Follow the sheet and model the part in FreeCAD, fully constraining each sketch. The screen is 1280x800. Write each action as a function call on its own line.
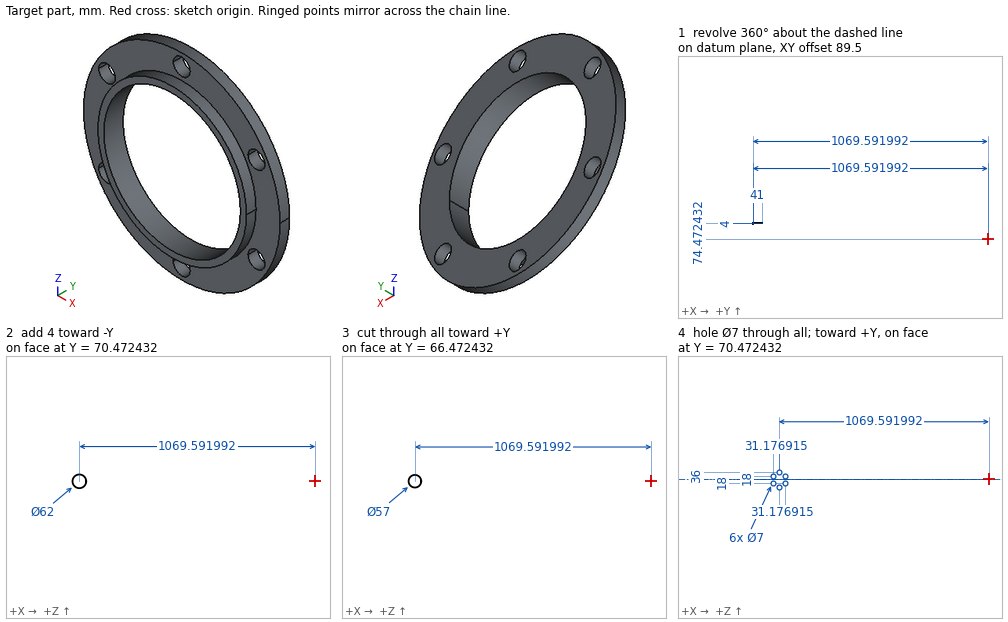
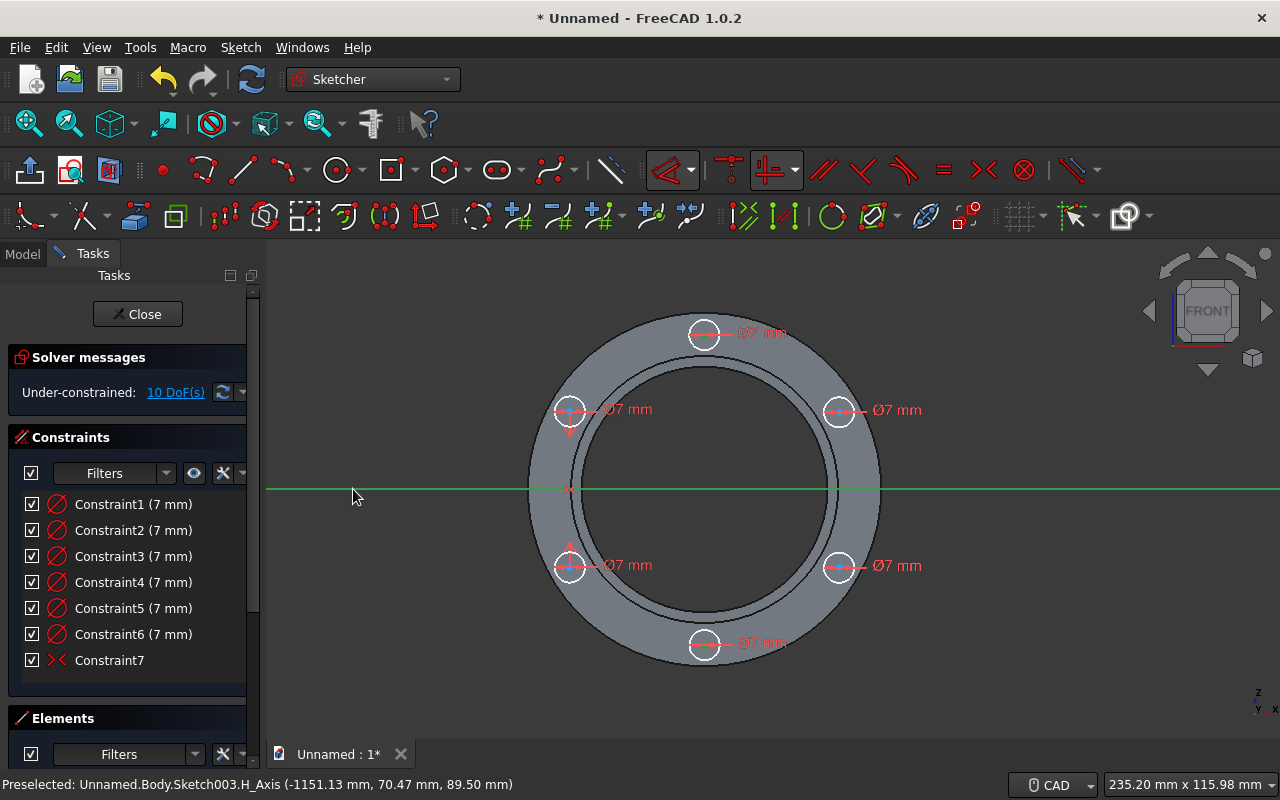
click(984, 170)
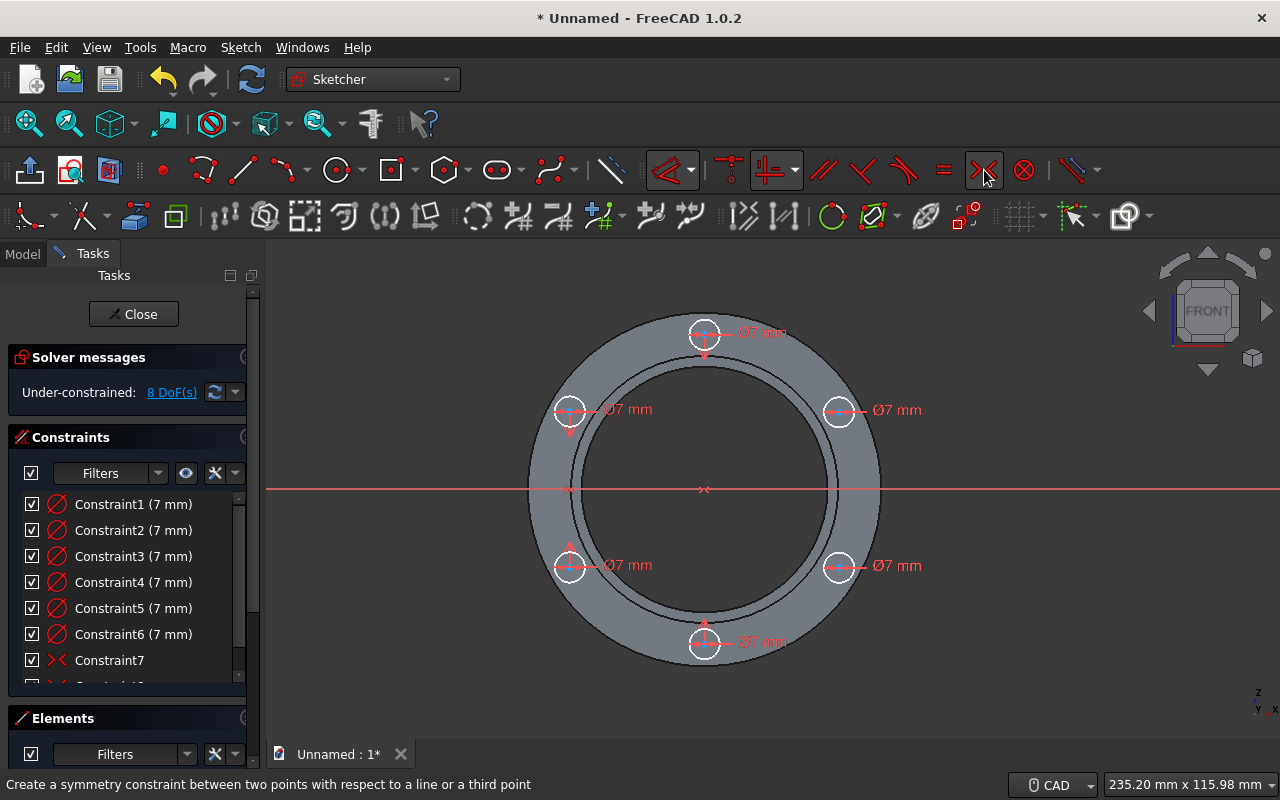
click(839, 568)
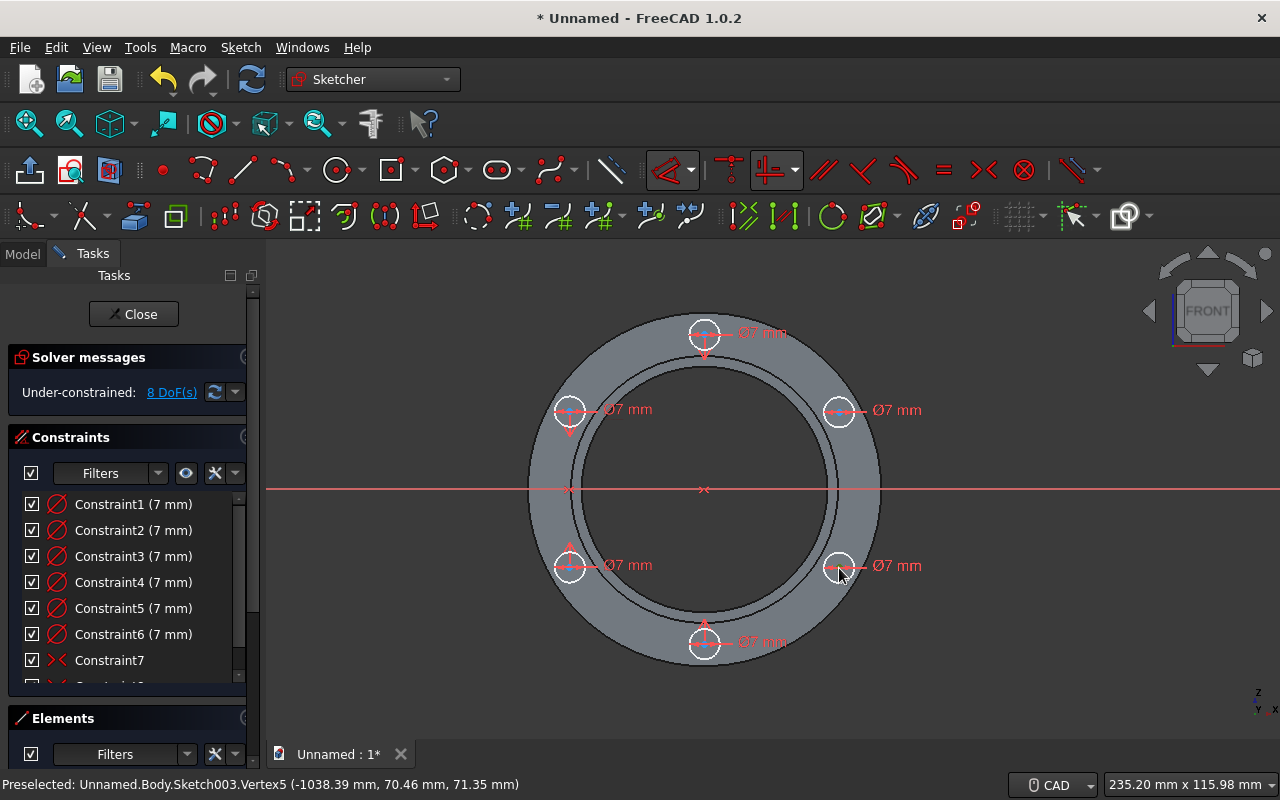
click(839, 412)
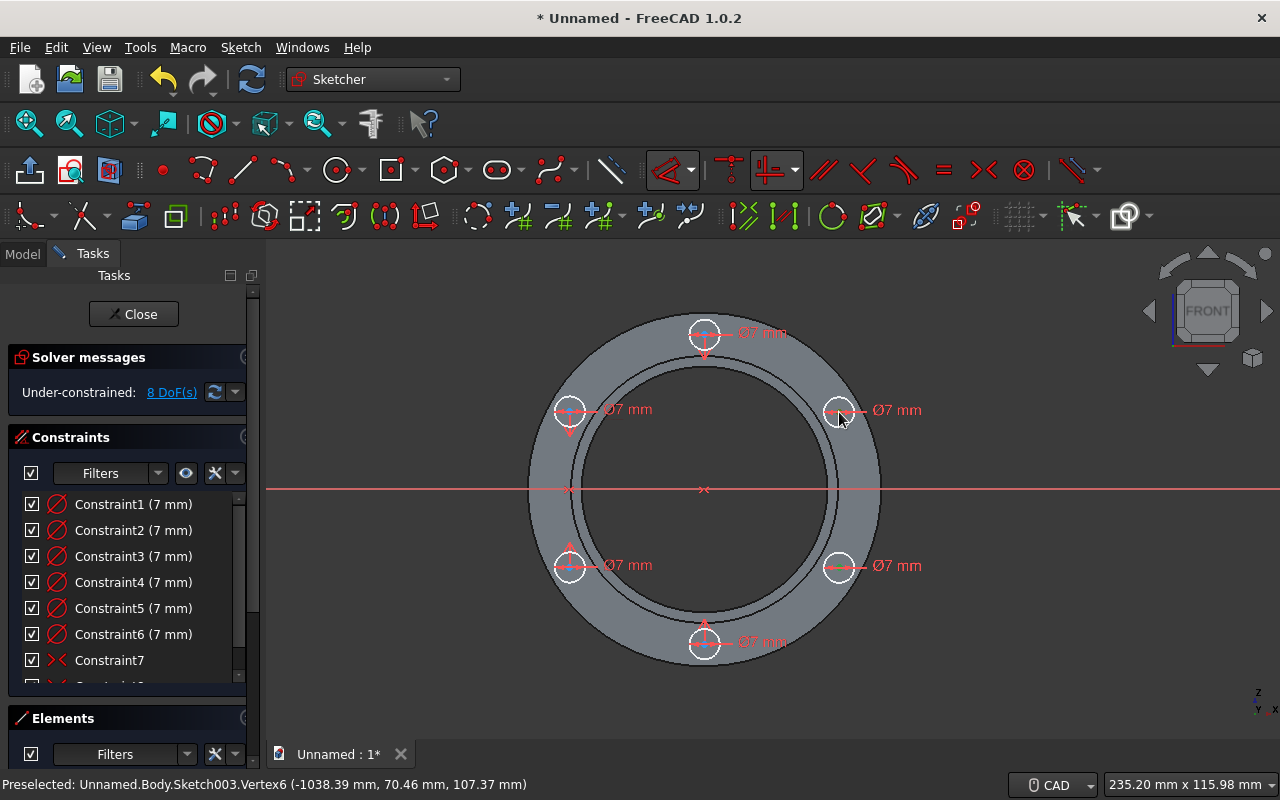
click(353, 489)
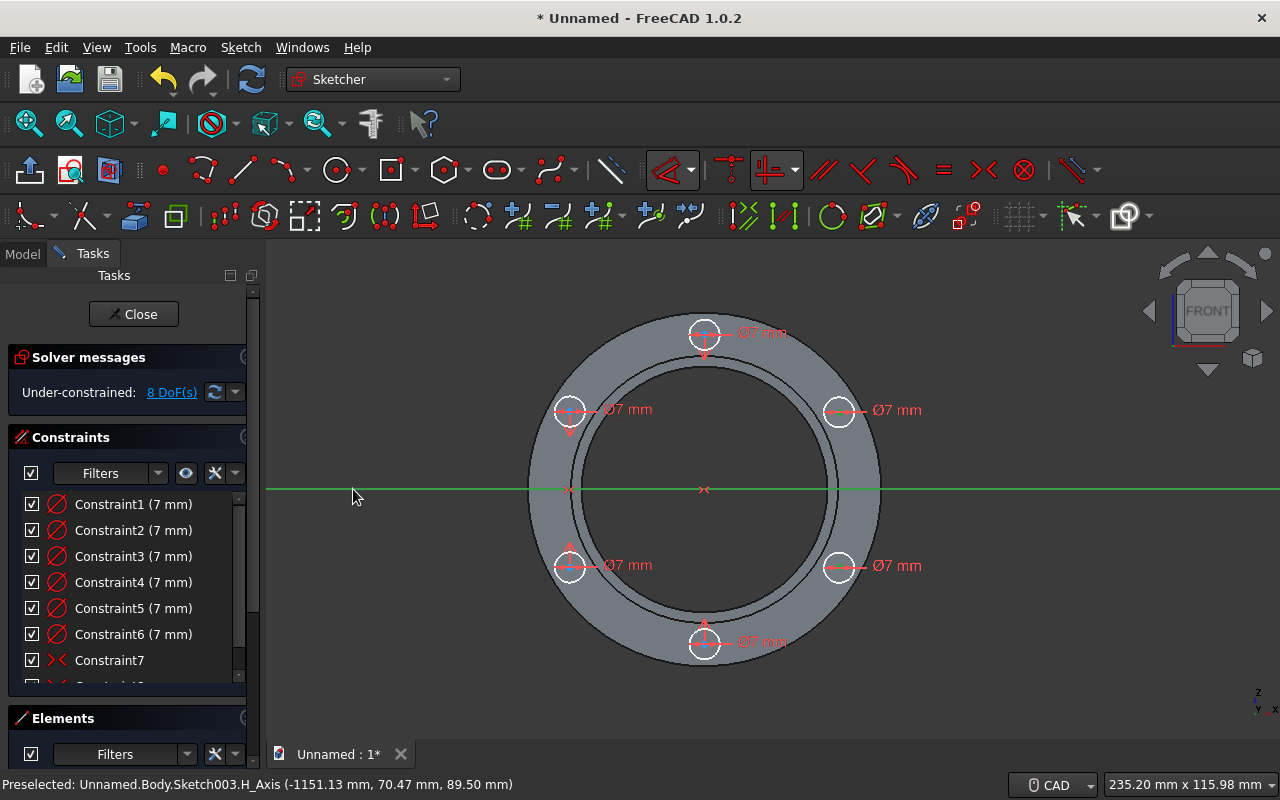
click(984, 170)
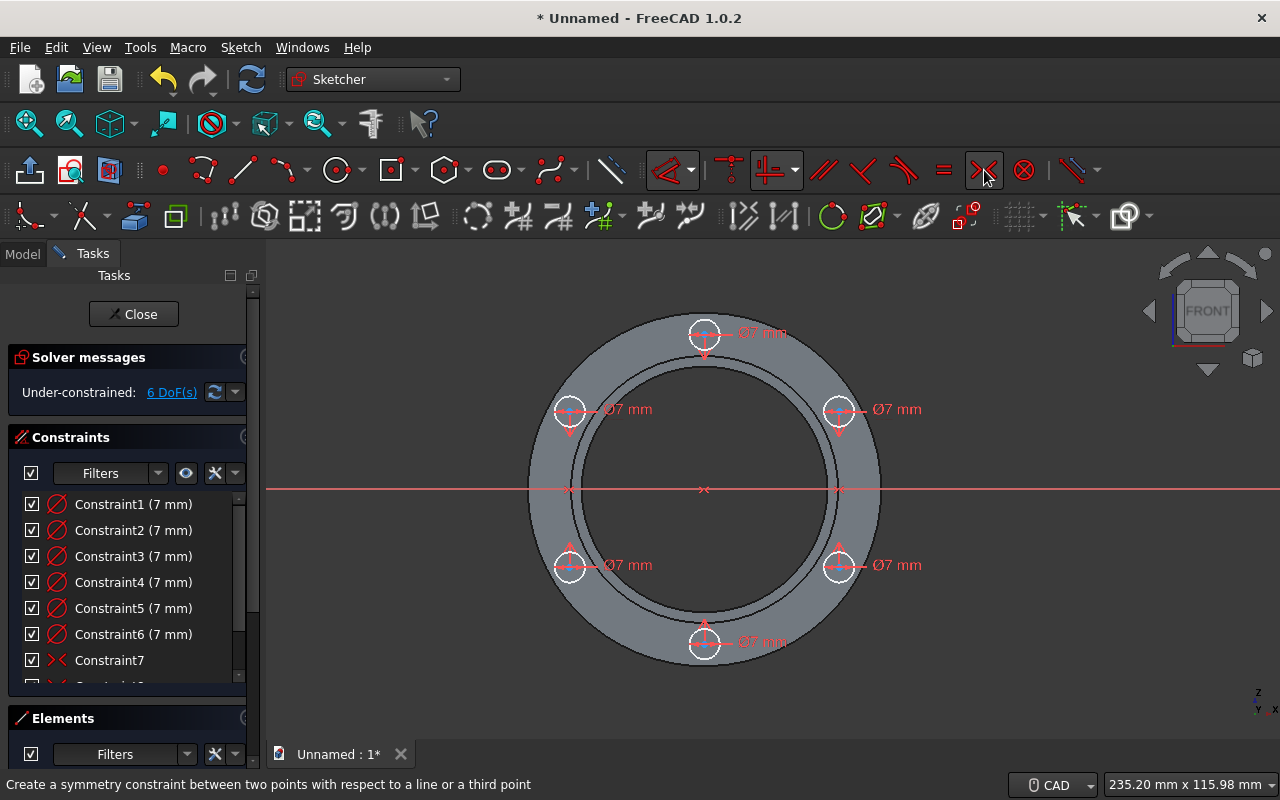
click(705, 335)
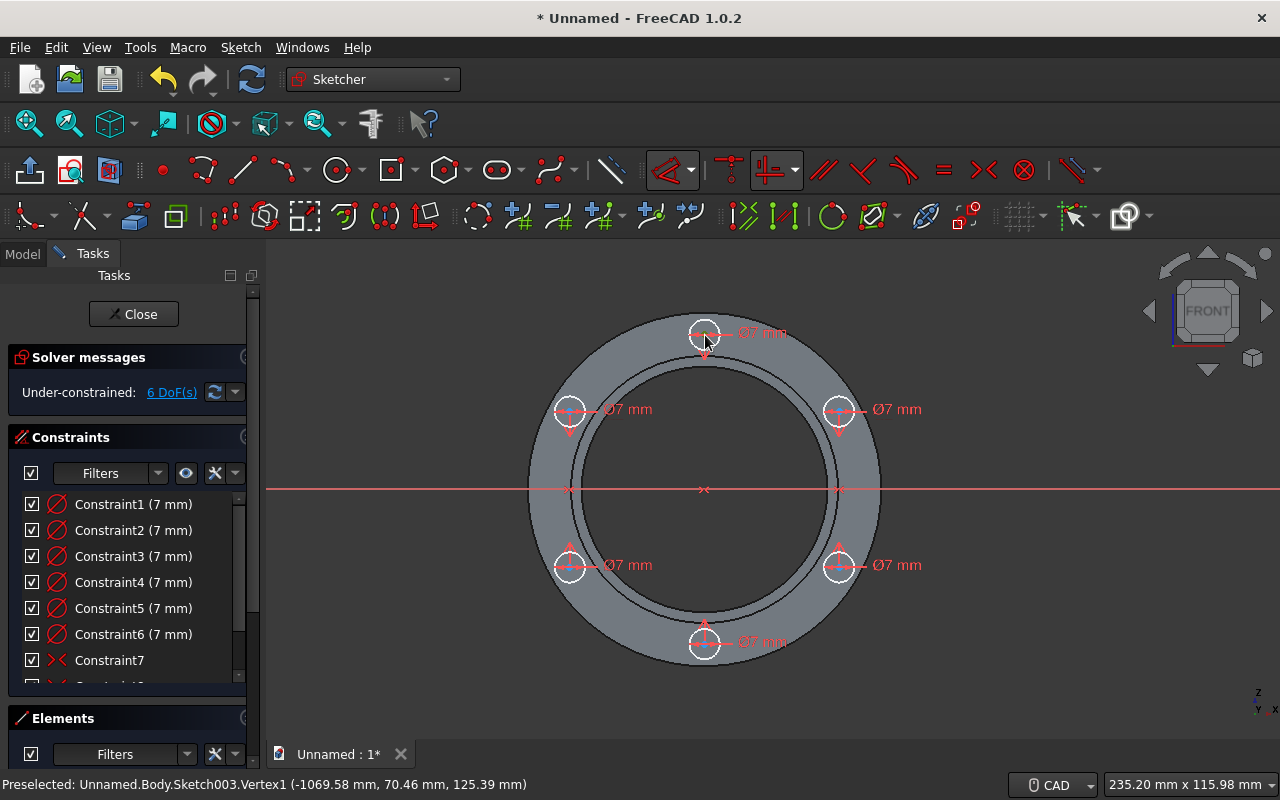
key(i)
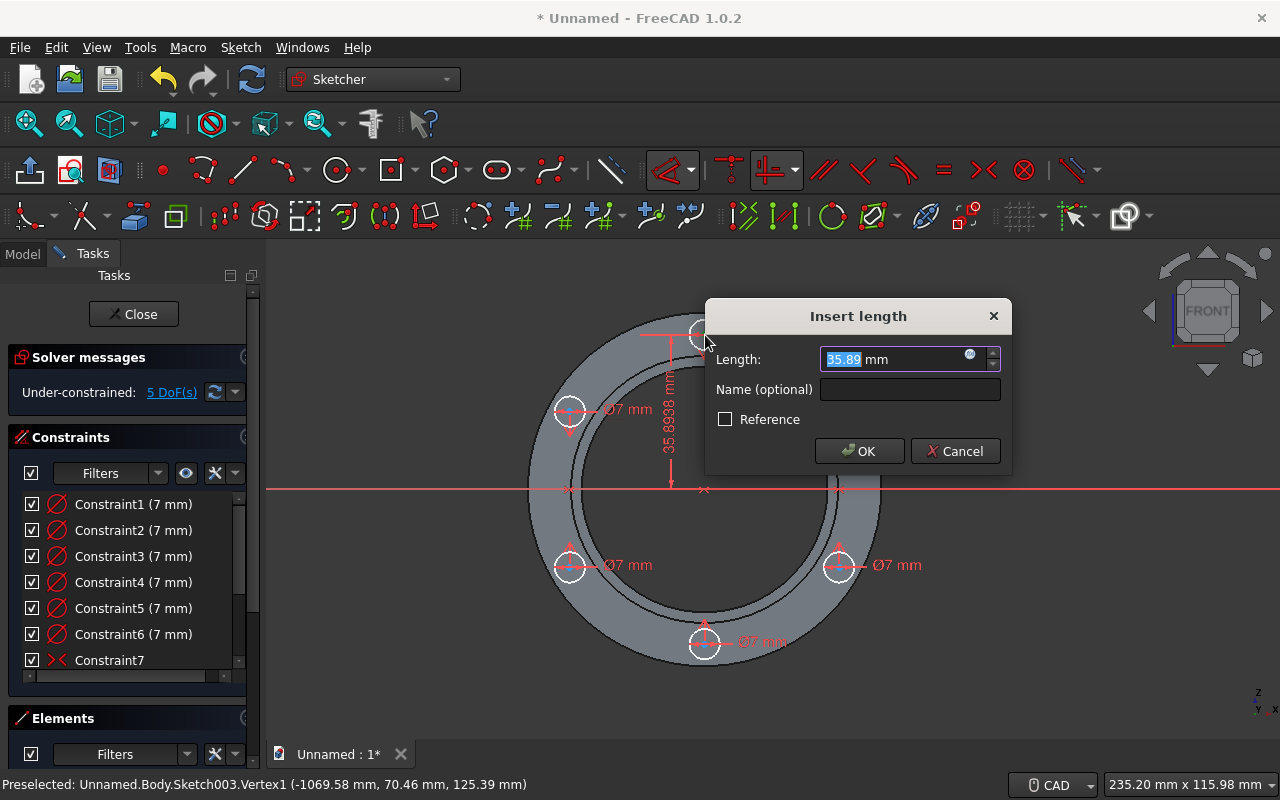
text(36)
key(Return)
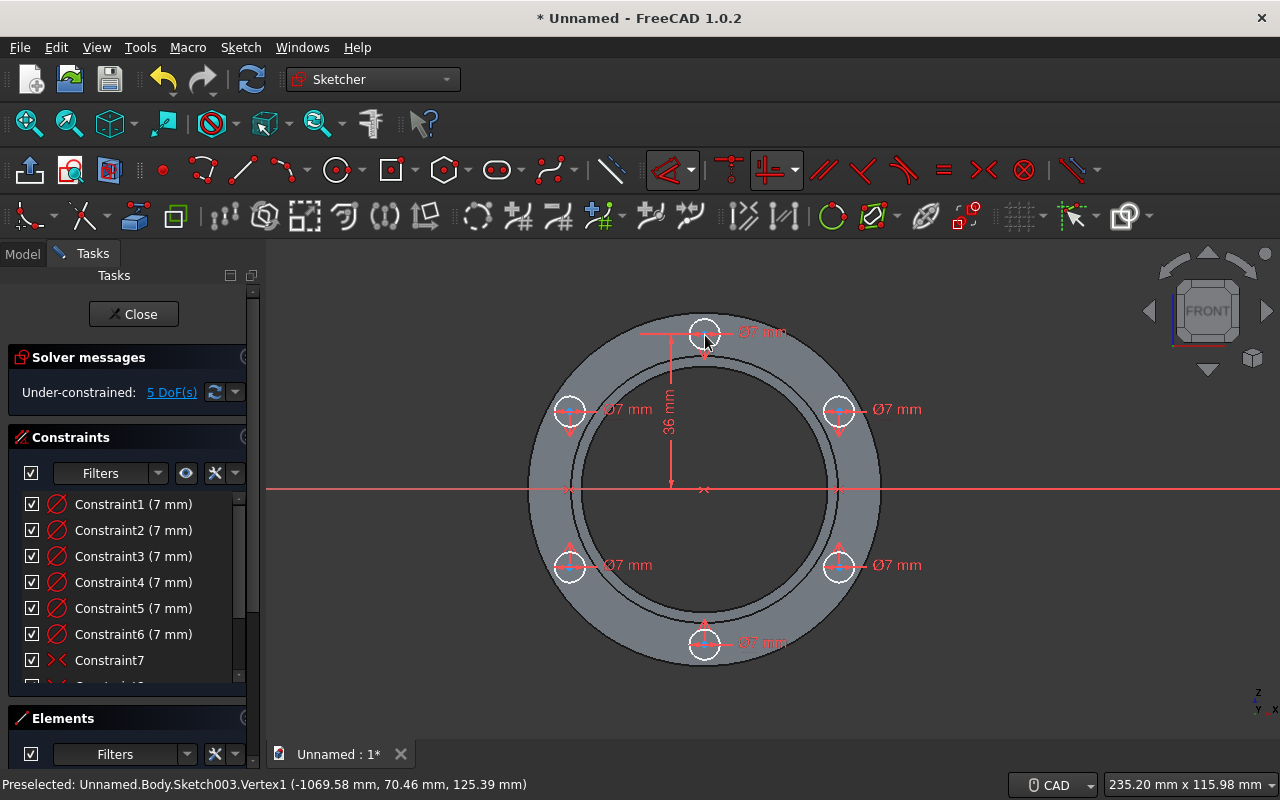
click(570, 412)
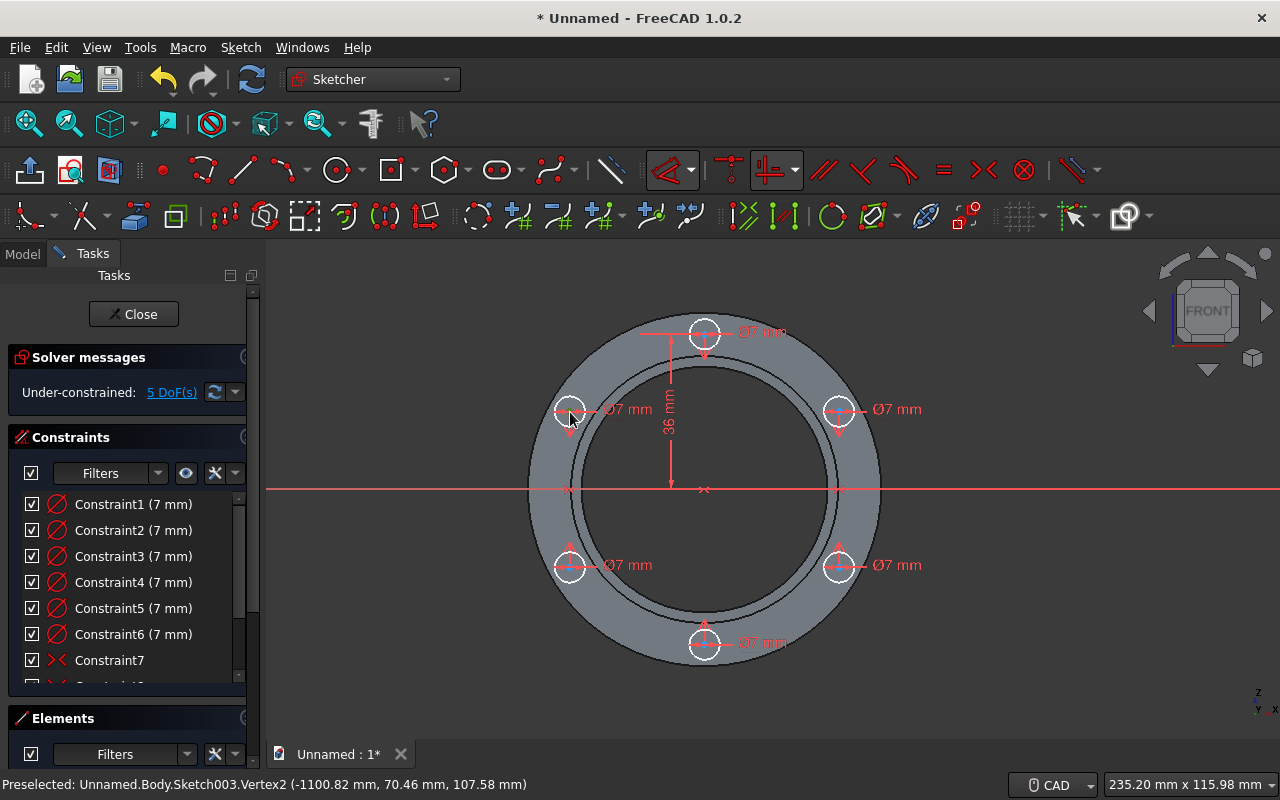
click(694, 170)